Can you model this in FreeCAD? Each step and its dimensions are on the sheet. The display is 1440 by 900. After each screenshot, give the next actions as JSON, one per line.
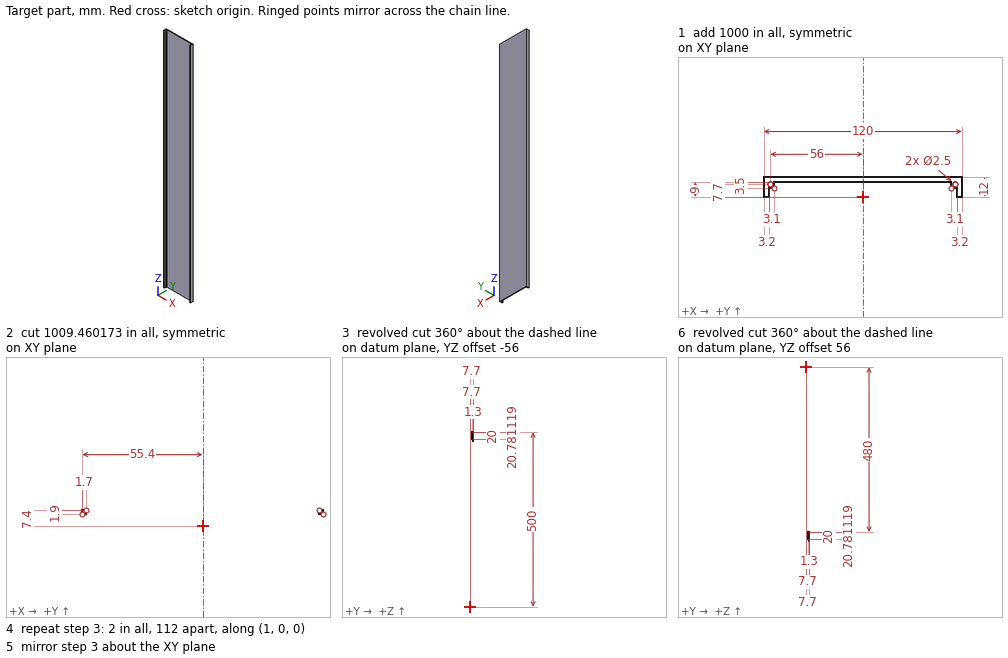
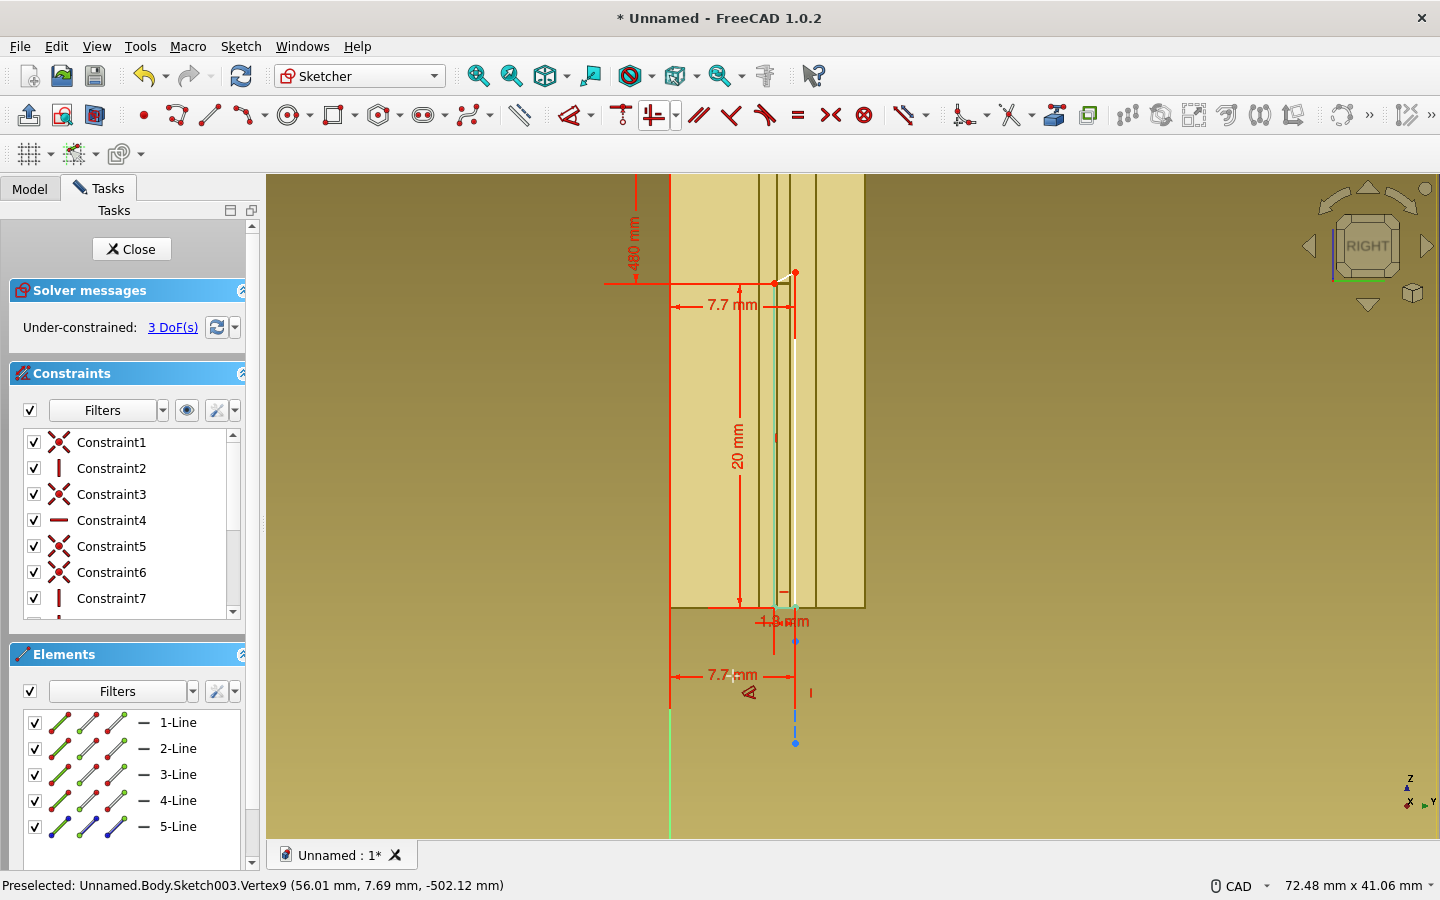
{"action": "left_click", "coordinate": [795, 507]}
{"action": "left_click", "coordinate": [829, 440]}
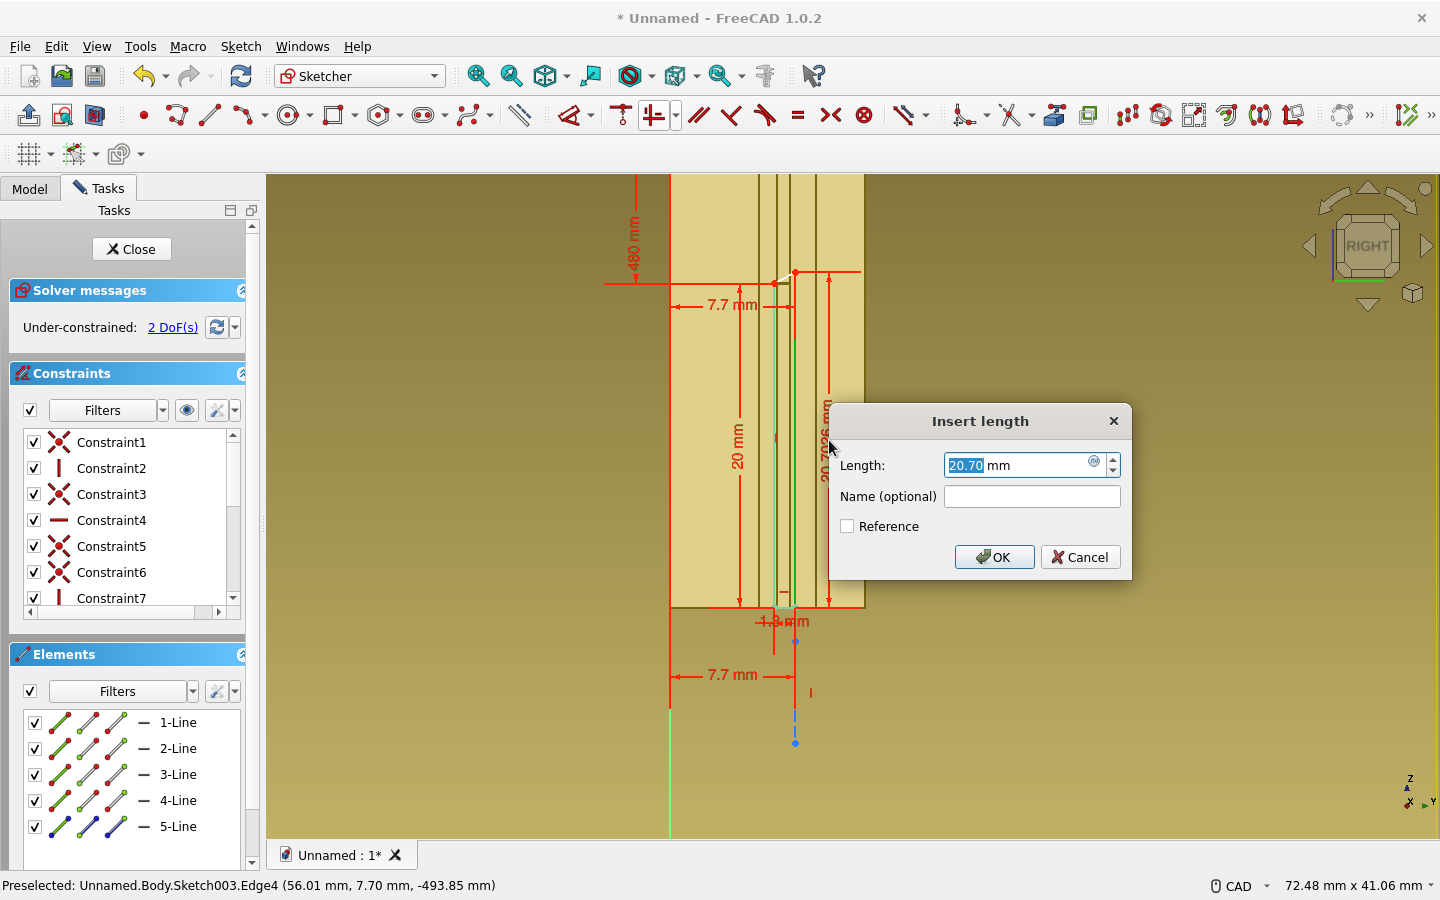
{"action": "type", "text": "20.781119"}
{"action": "key", "text": "Return"}
{"action": "key", "text": "Escape"}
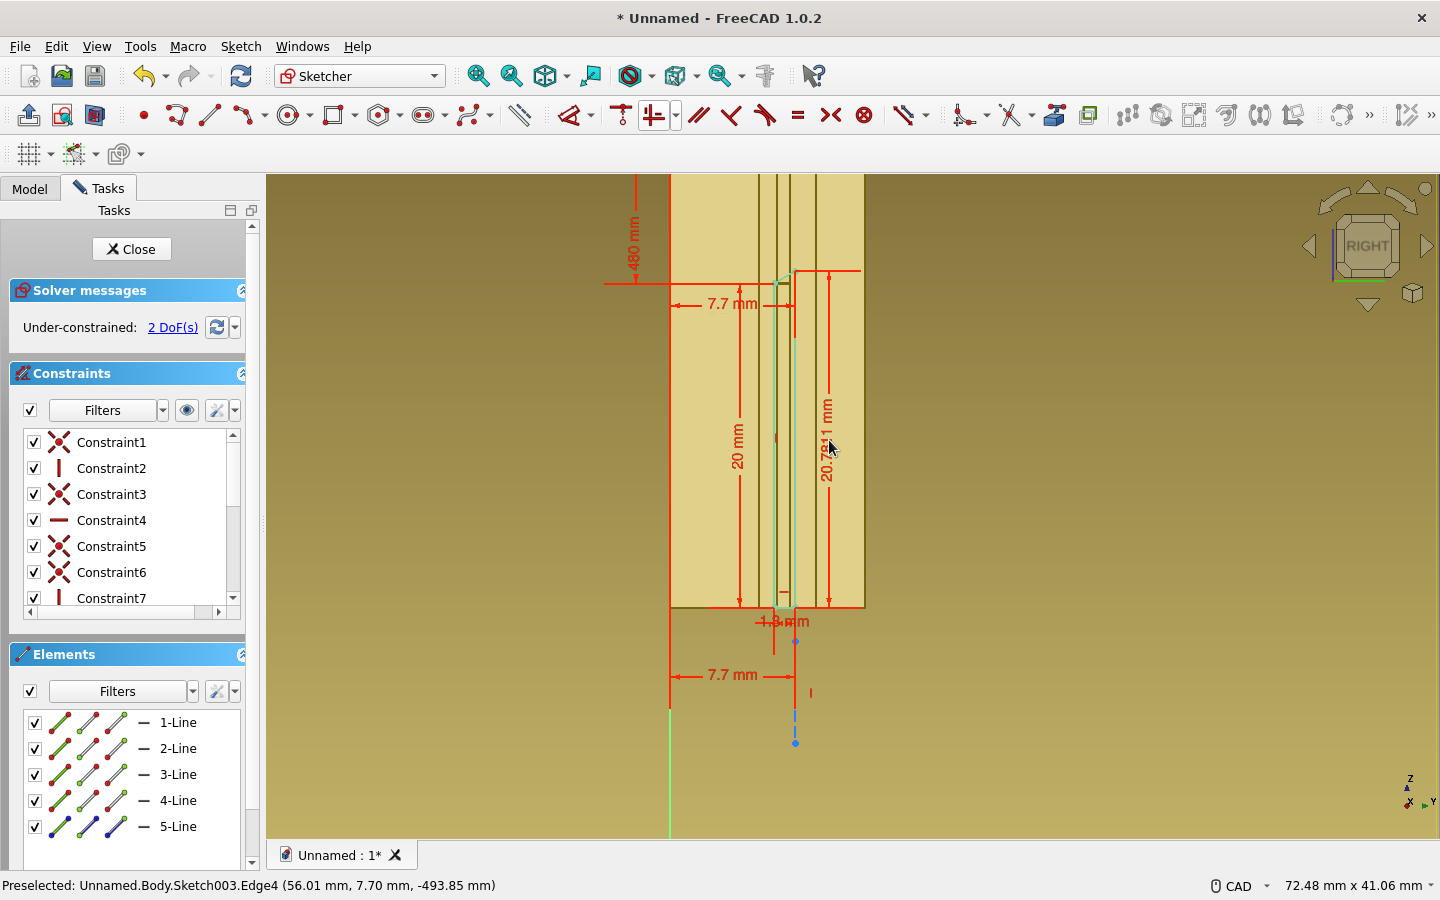
{"action": "left_click", "coordinate": [132, 249]}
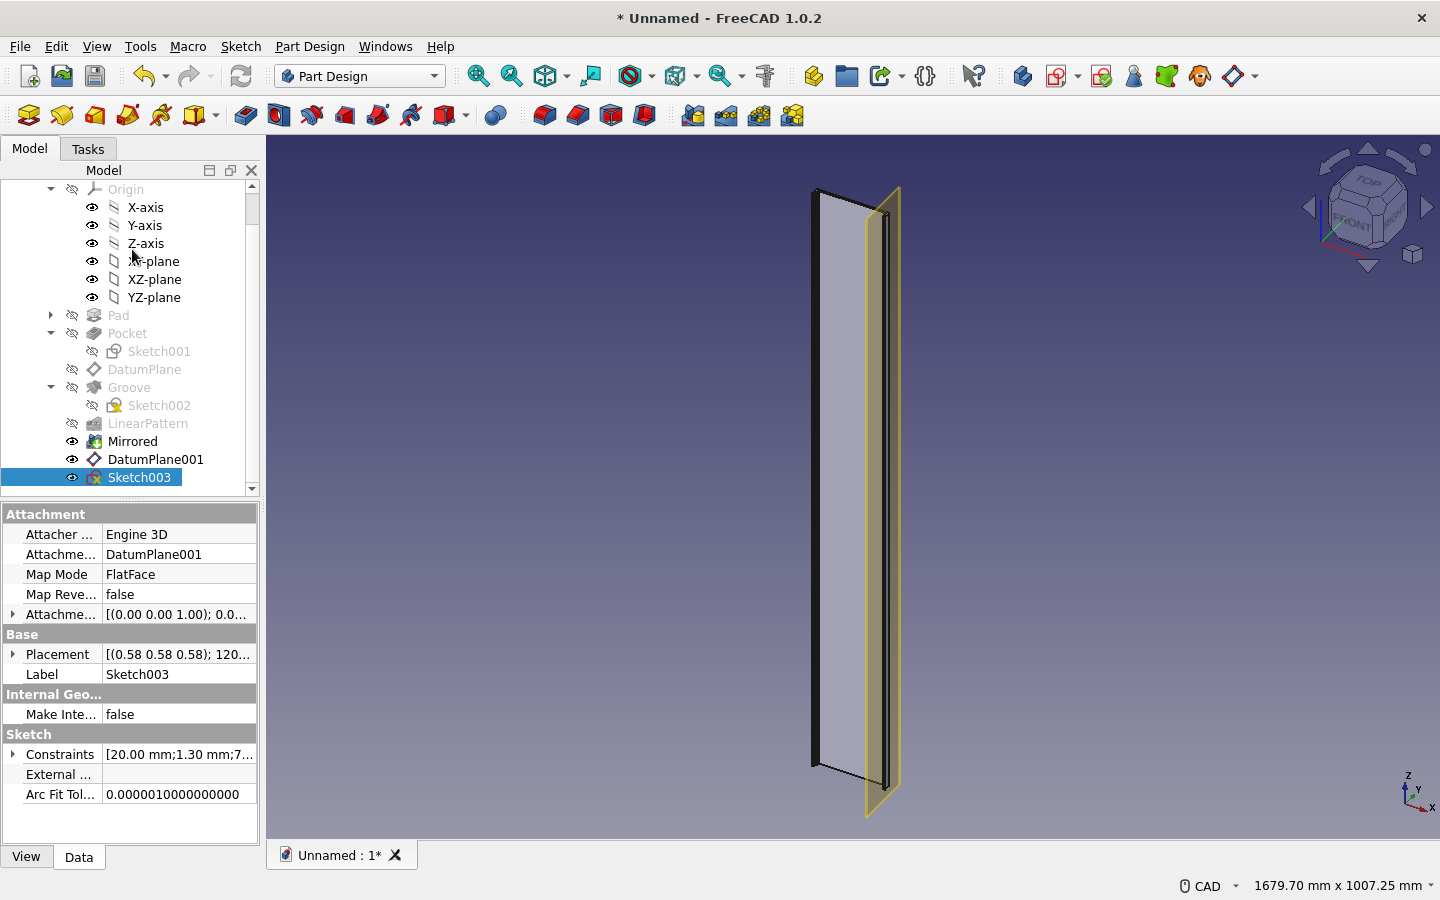
{"action": "left_click", "coordinate": [312, 116]}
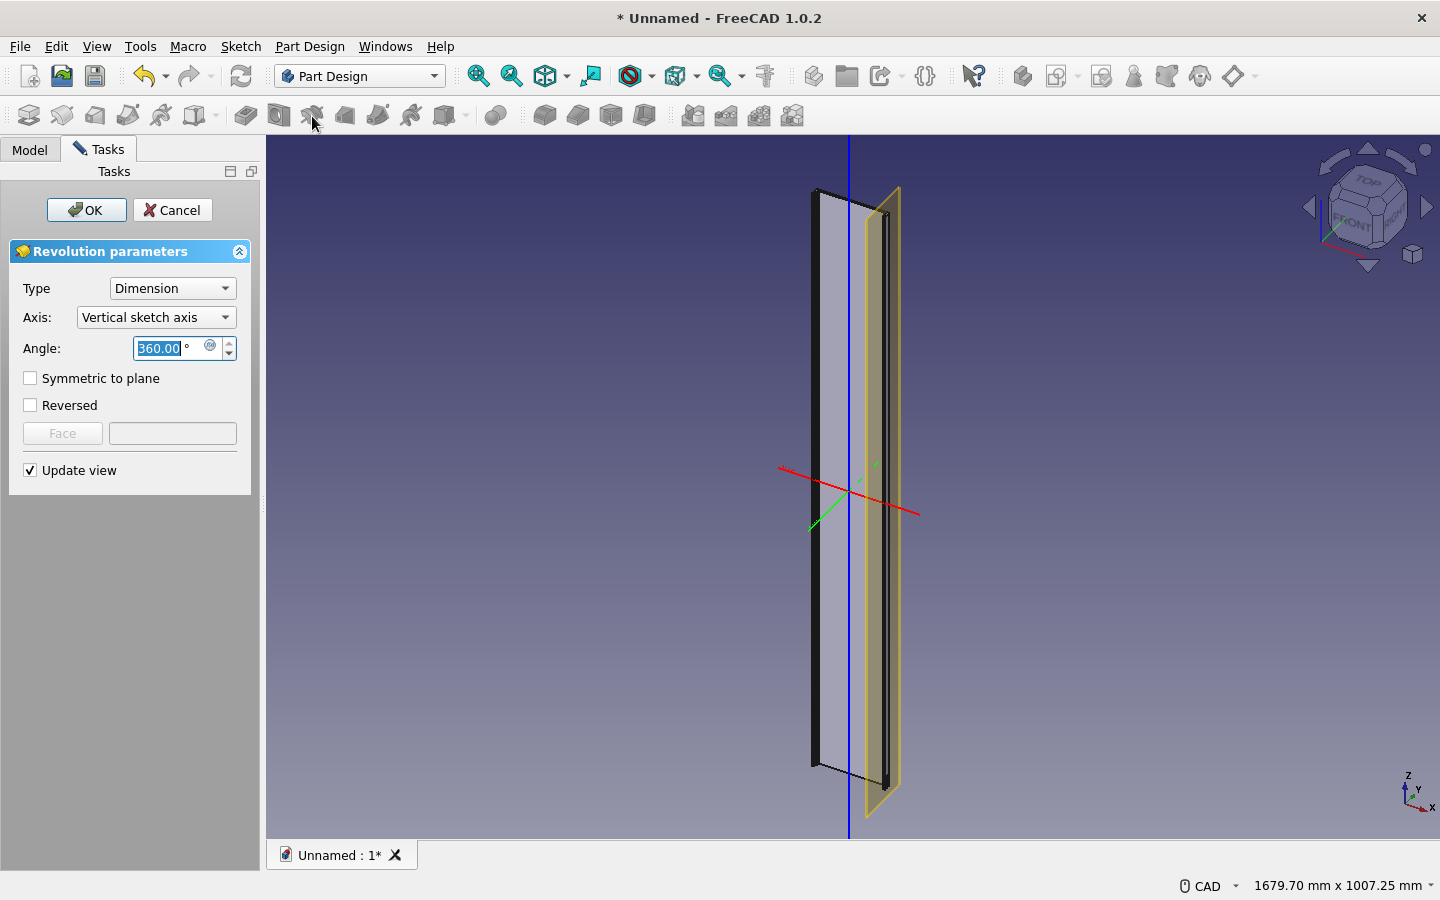
{"action": "left_click", "coordinate": [157, 318]}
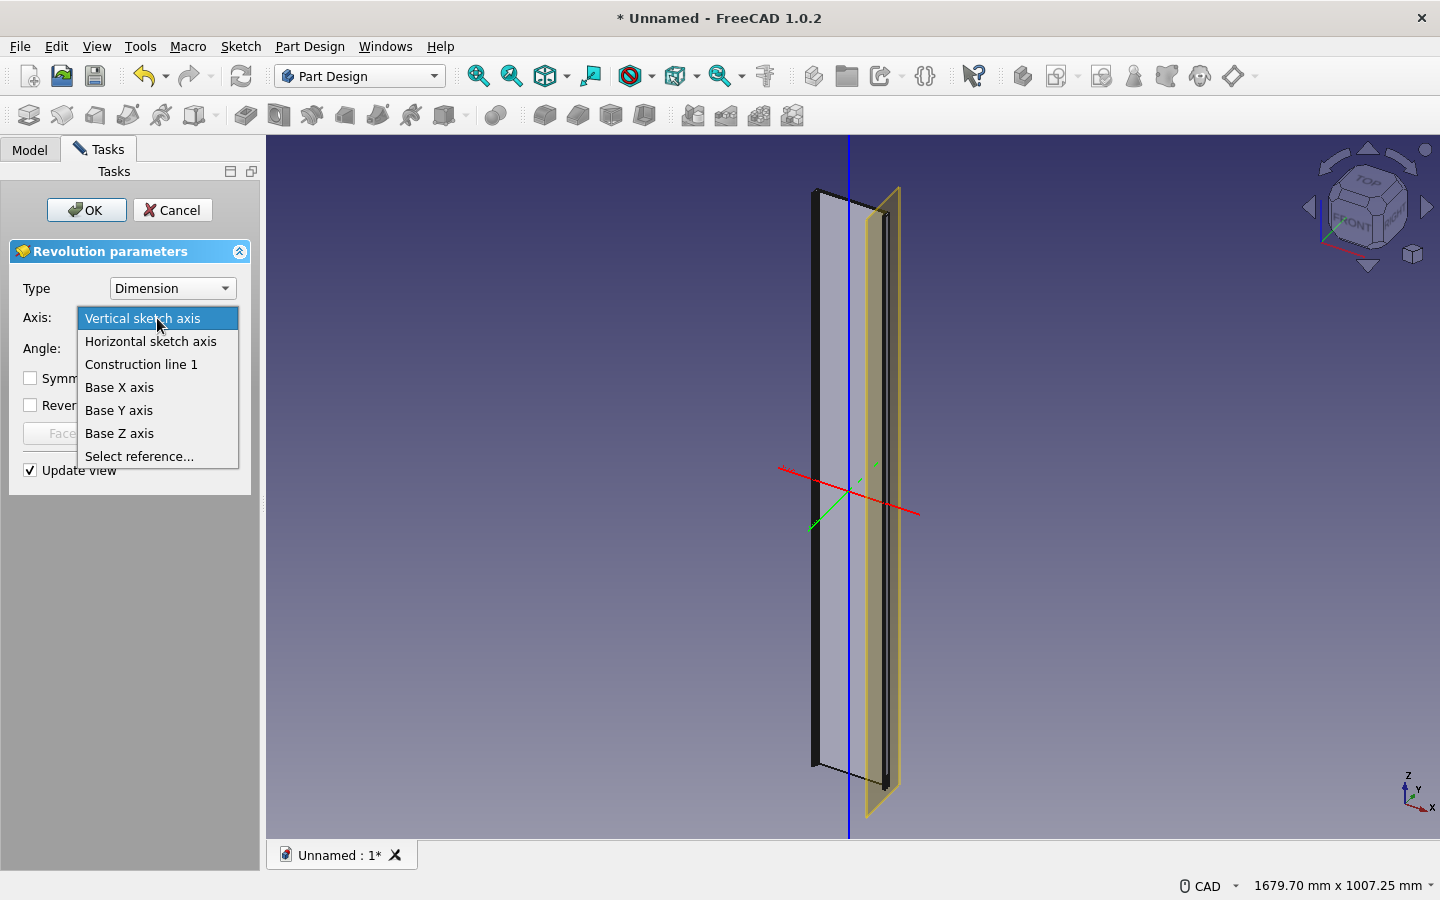
{"action": "left_click", "coordinate": [156, 364]}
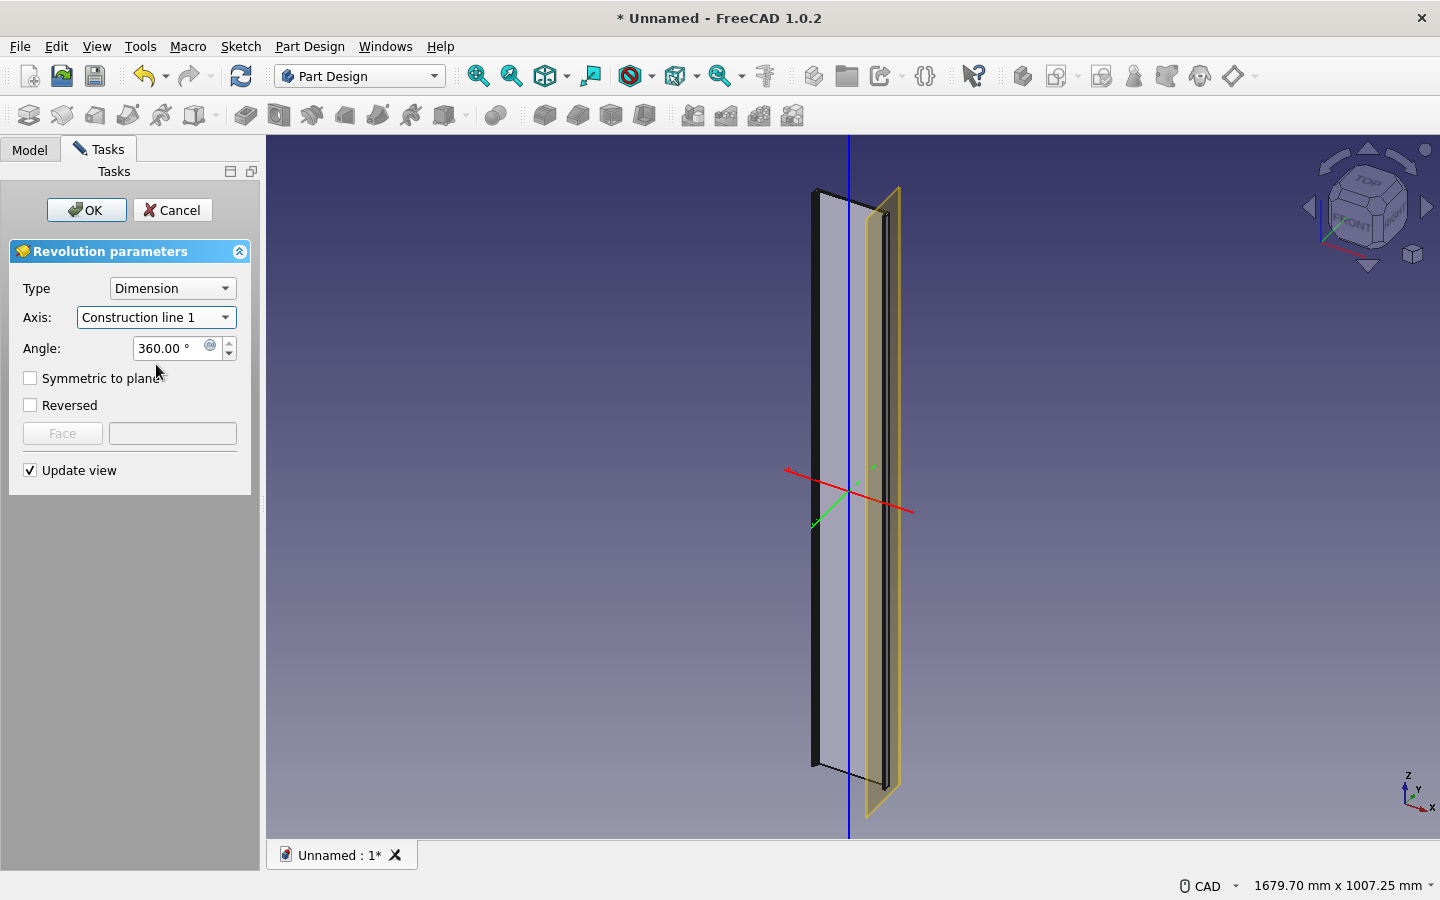
{"action": "left_click", "coordinate": [87, 210]}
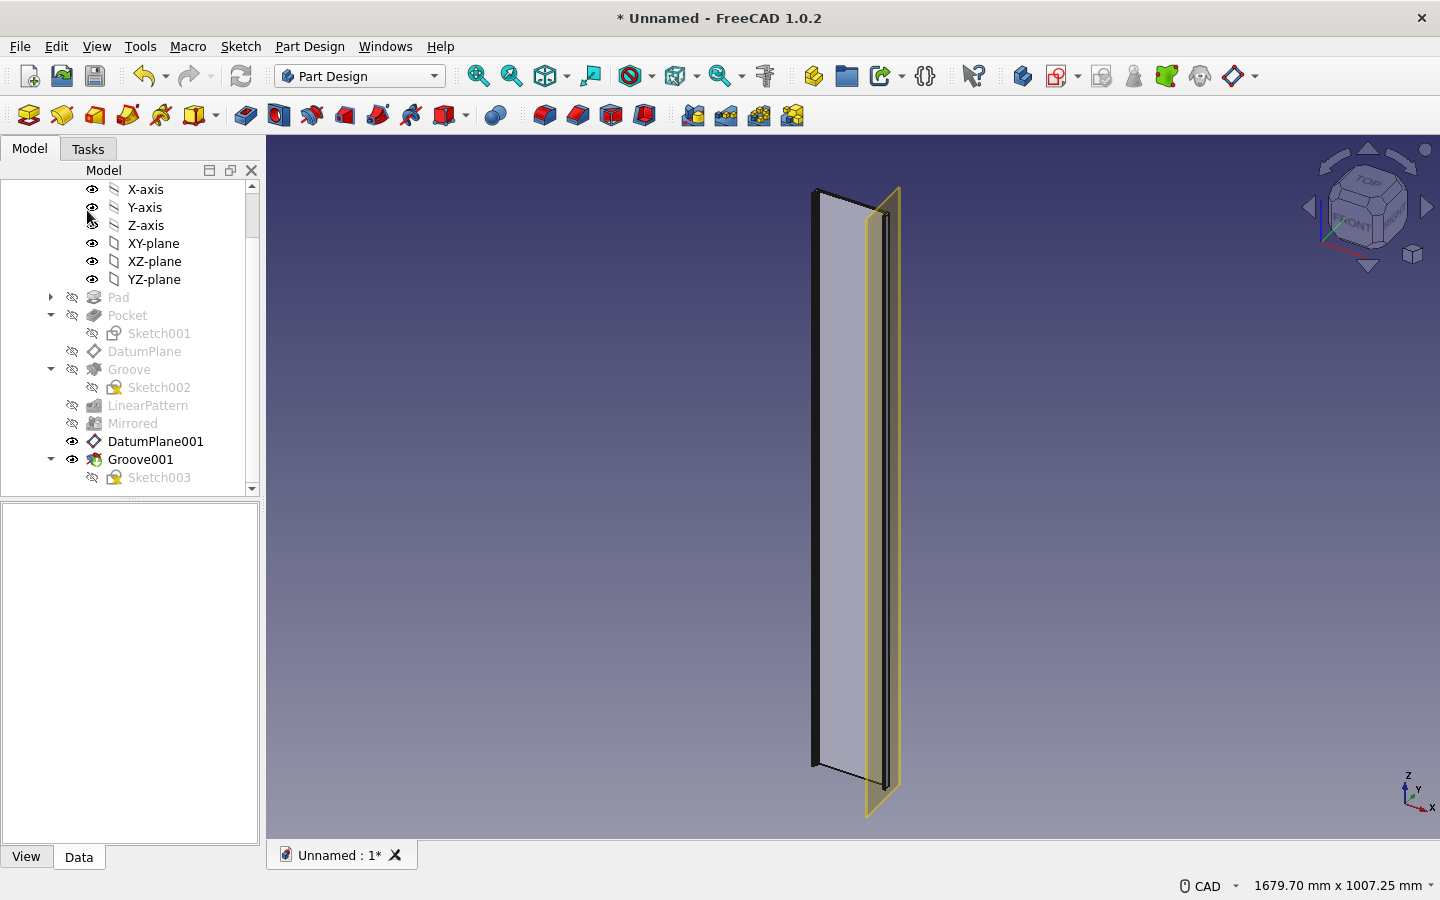
{"action": "left_click", "coordinate": [117, 441]}
{"action": "key", "text": "space"}